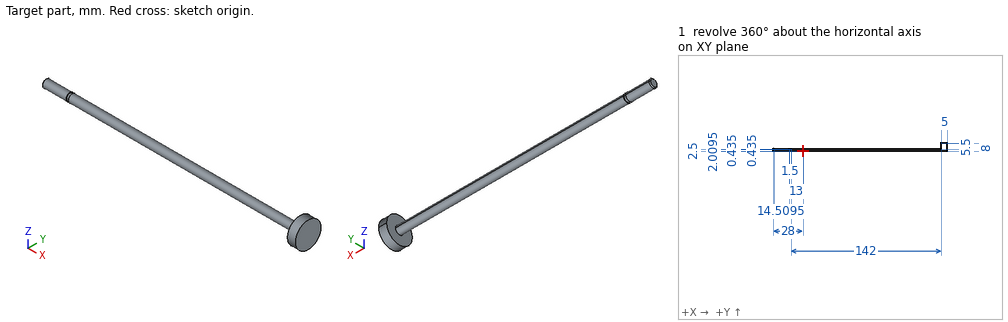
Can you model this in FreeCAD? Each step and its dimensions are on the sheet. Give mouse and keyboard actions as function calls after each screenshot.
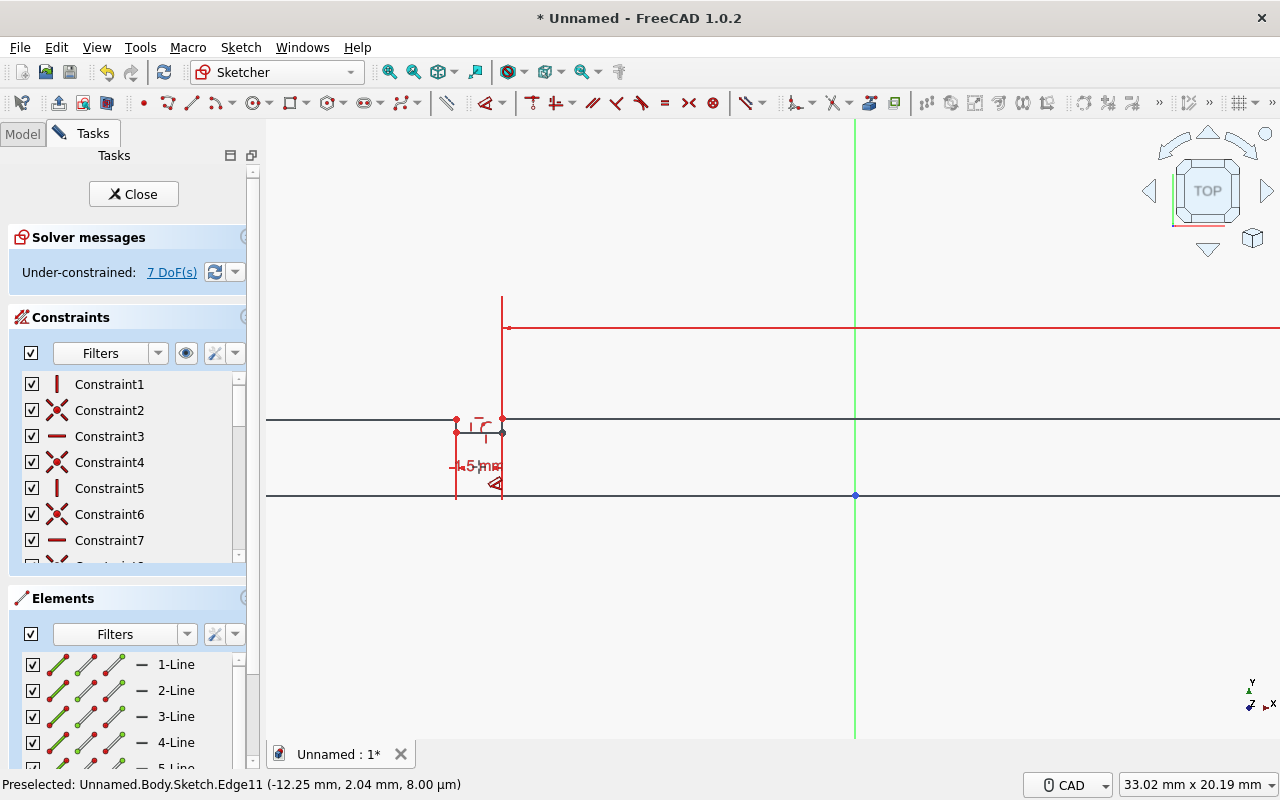
scroll(480, 436, down, 11)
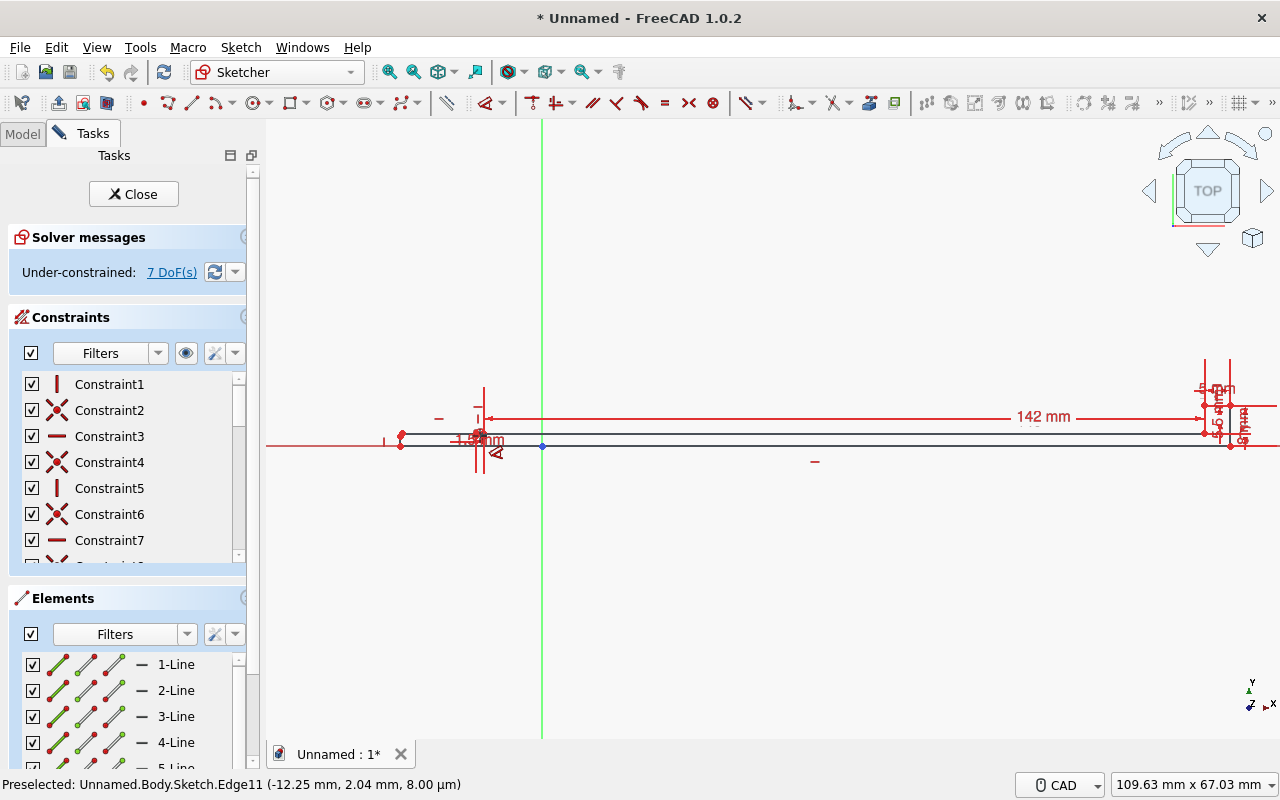
scroll(427, 443, up, 4)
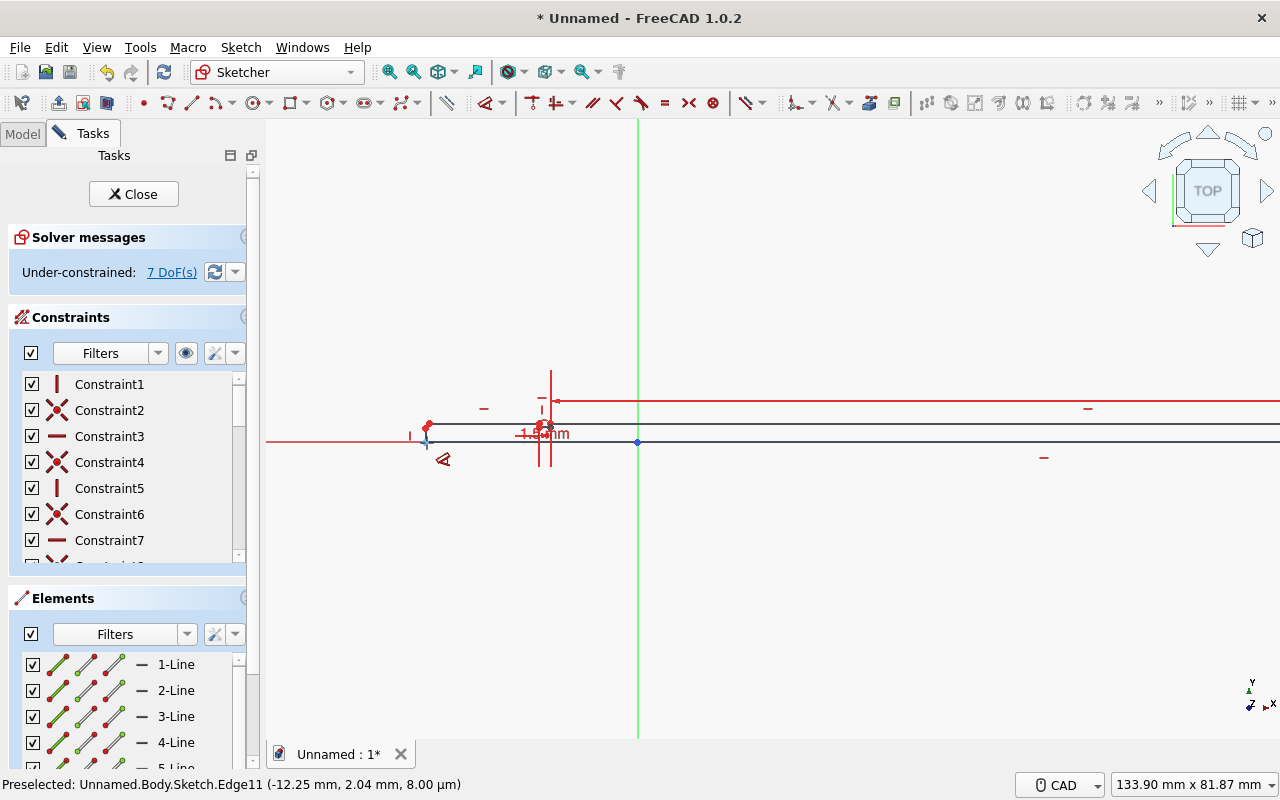
click(426, 442)
click(532, 476)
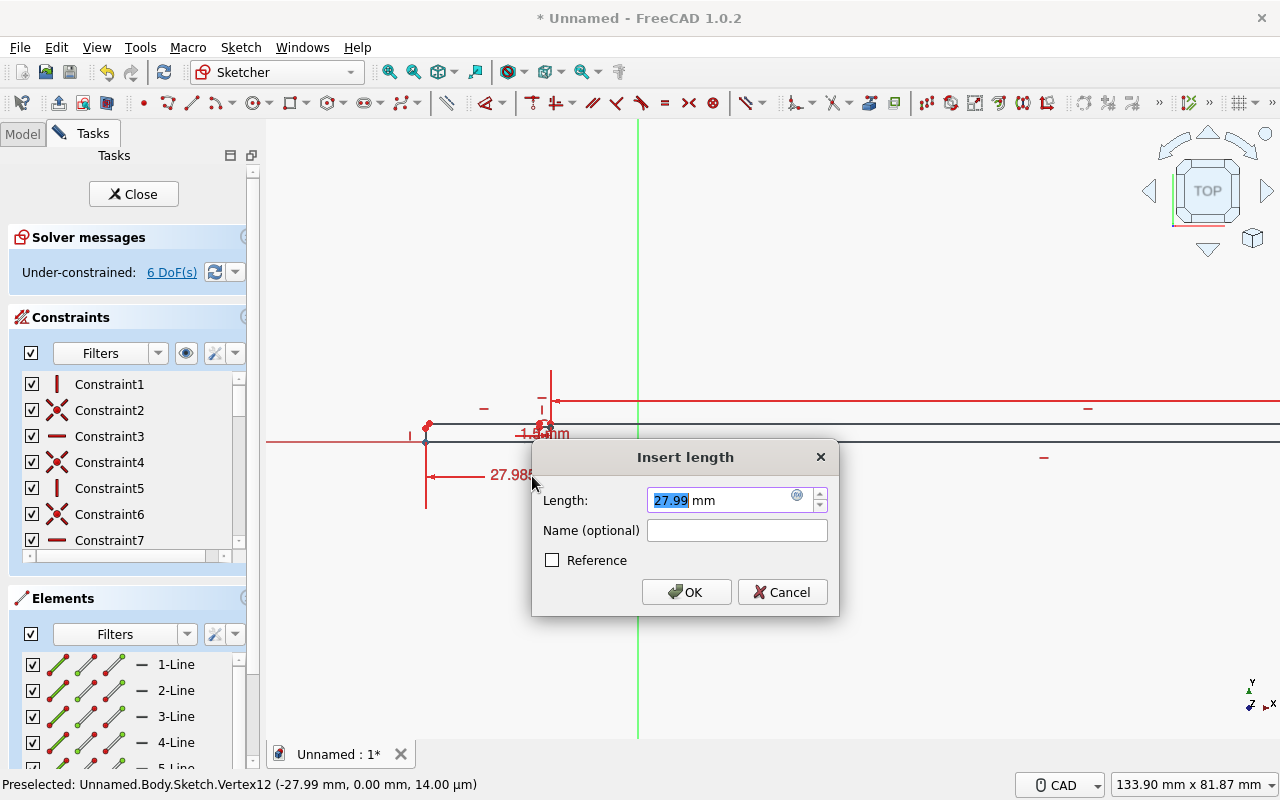
text(28)
key(Return)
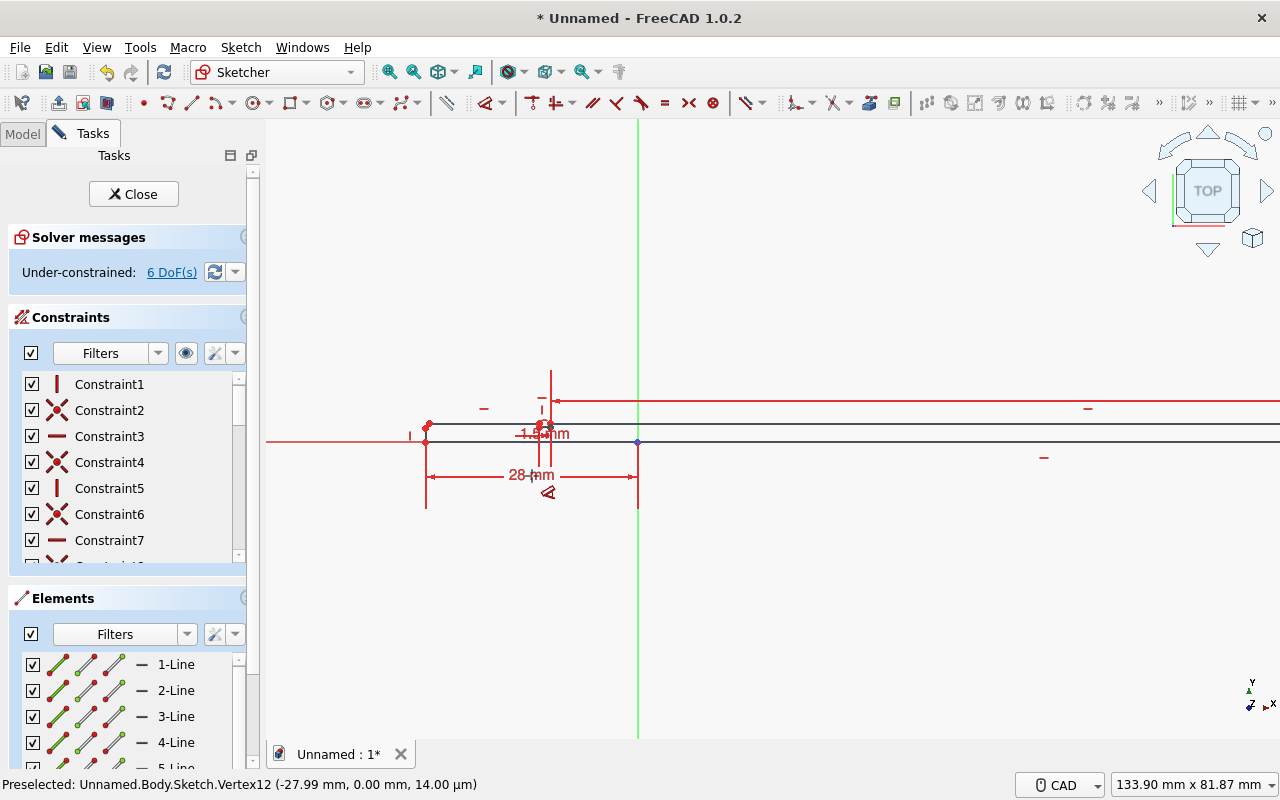
scroll(539, 424, up, 7)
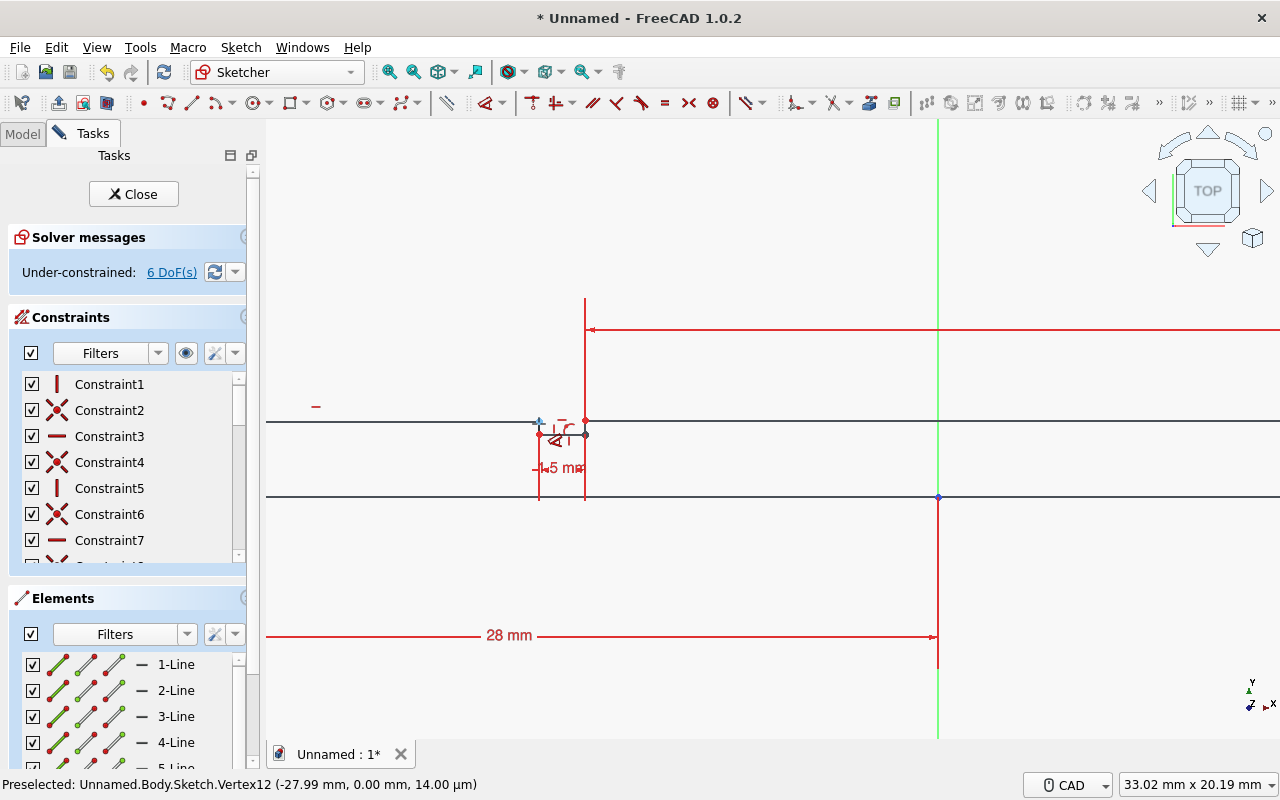
click(539, 422)
click(739, 531)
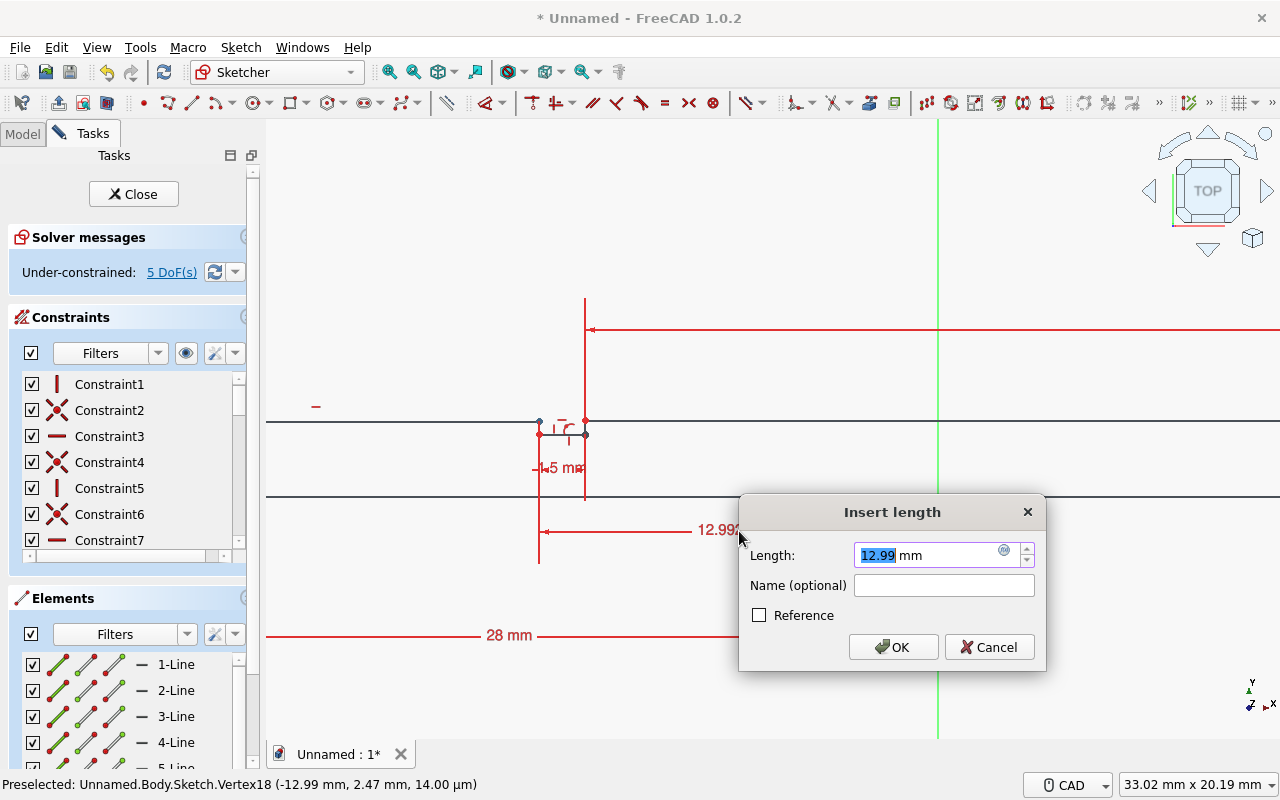
text(13)
key(Return)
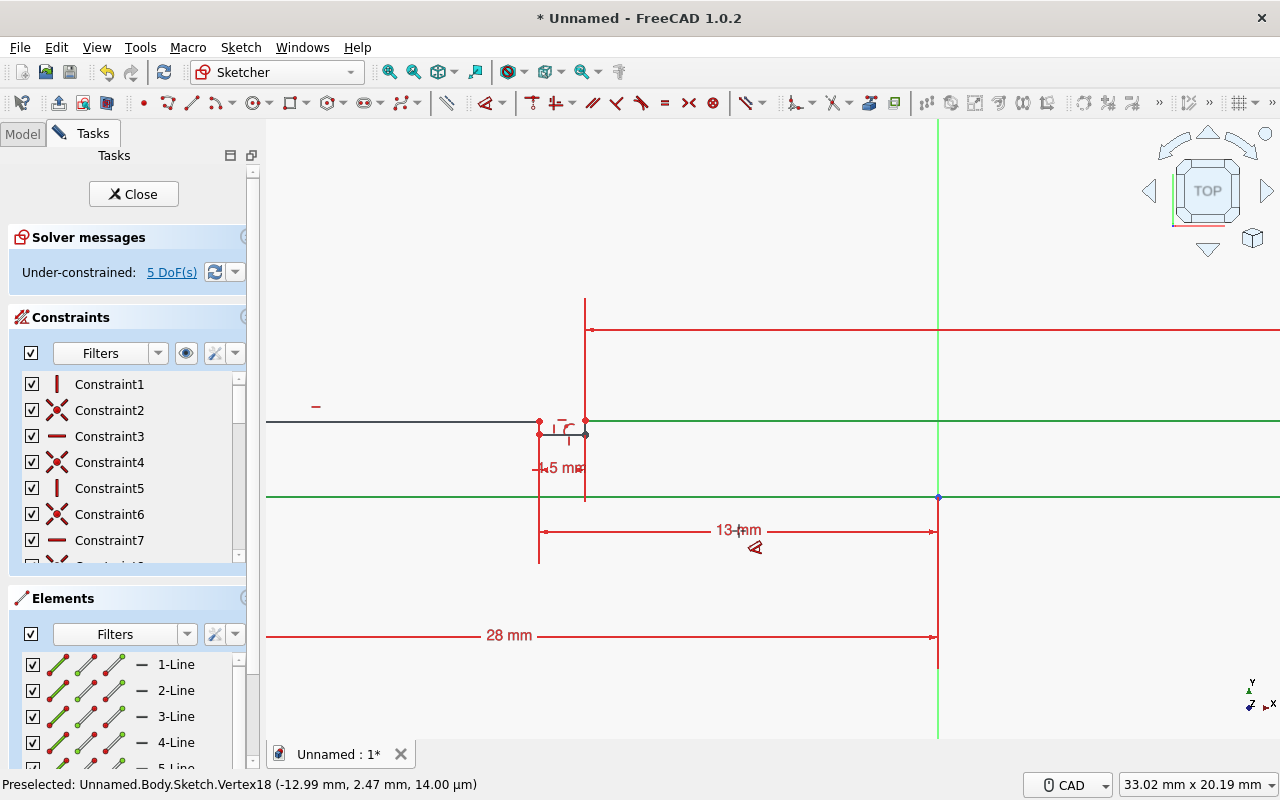
scroll(470, 436, down, 11)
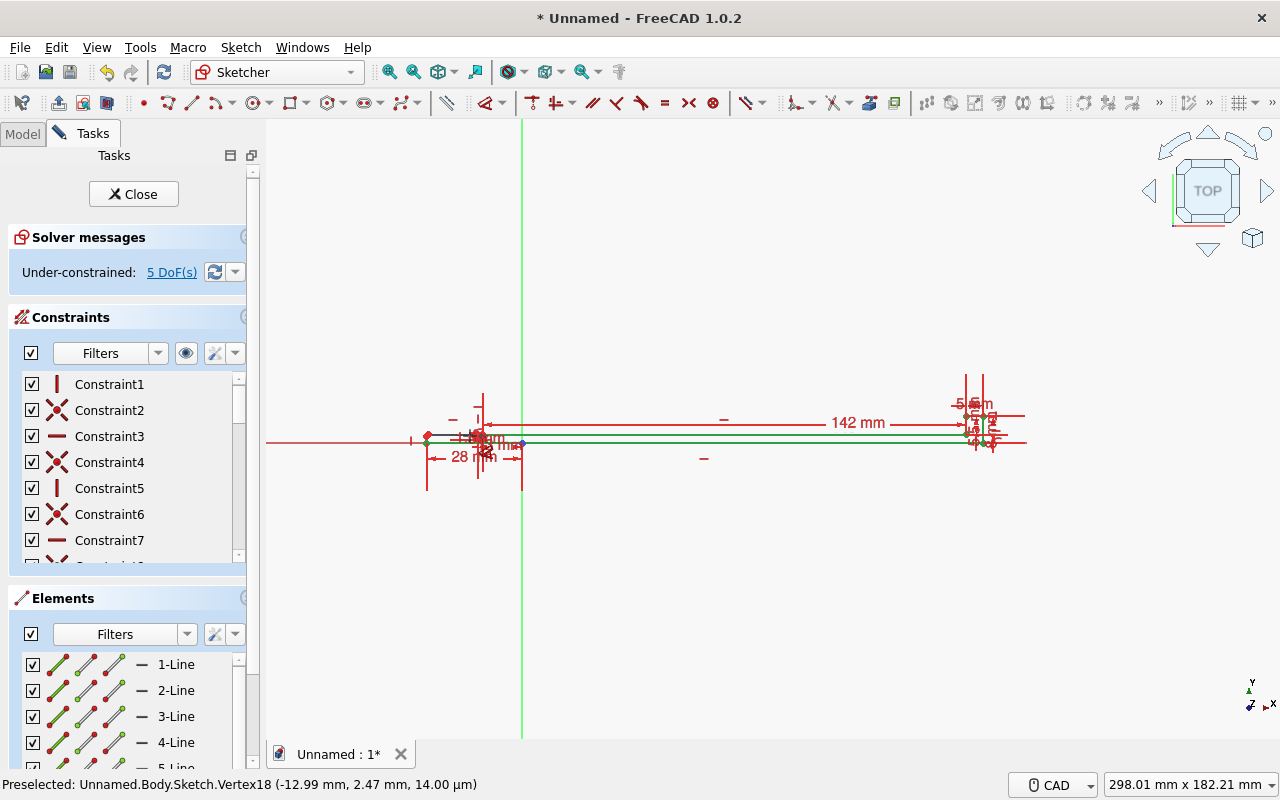
scroll(428, 435, up, 8)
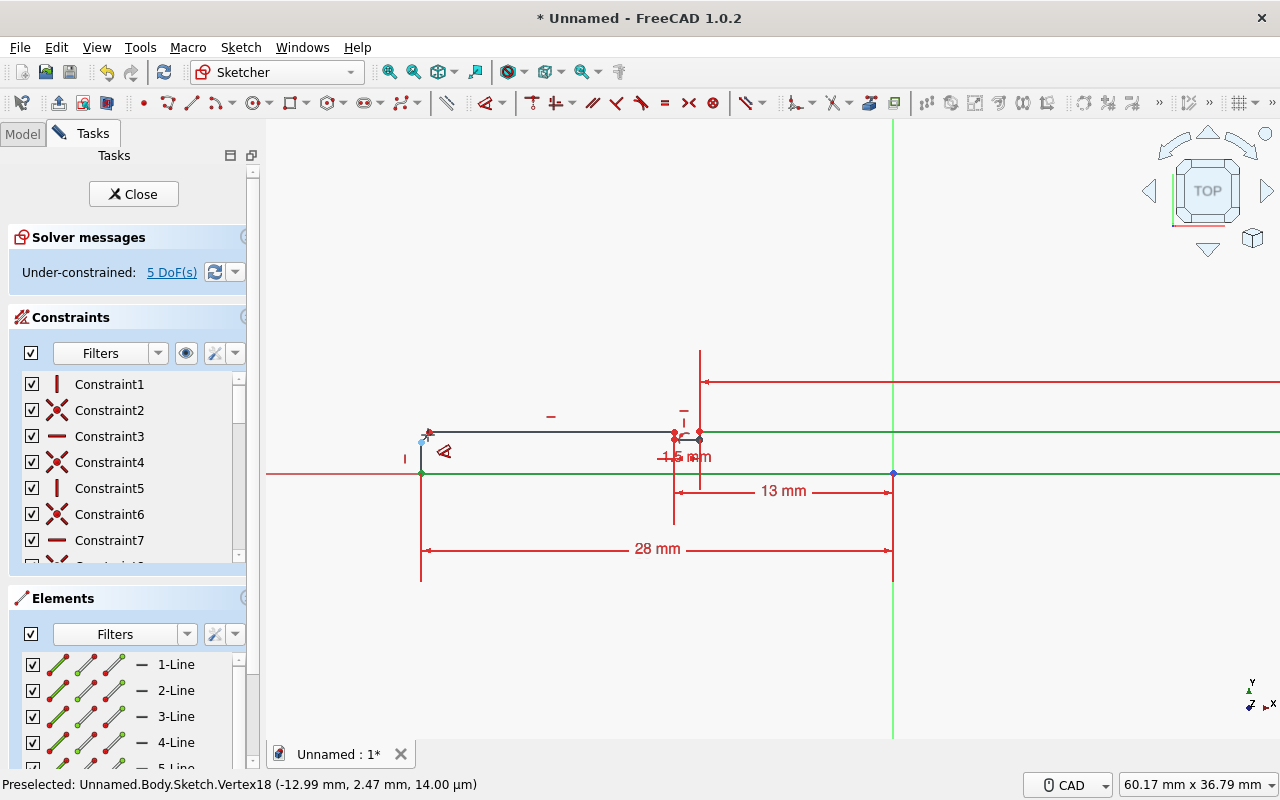
click(430, 432)
click(396, 453)